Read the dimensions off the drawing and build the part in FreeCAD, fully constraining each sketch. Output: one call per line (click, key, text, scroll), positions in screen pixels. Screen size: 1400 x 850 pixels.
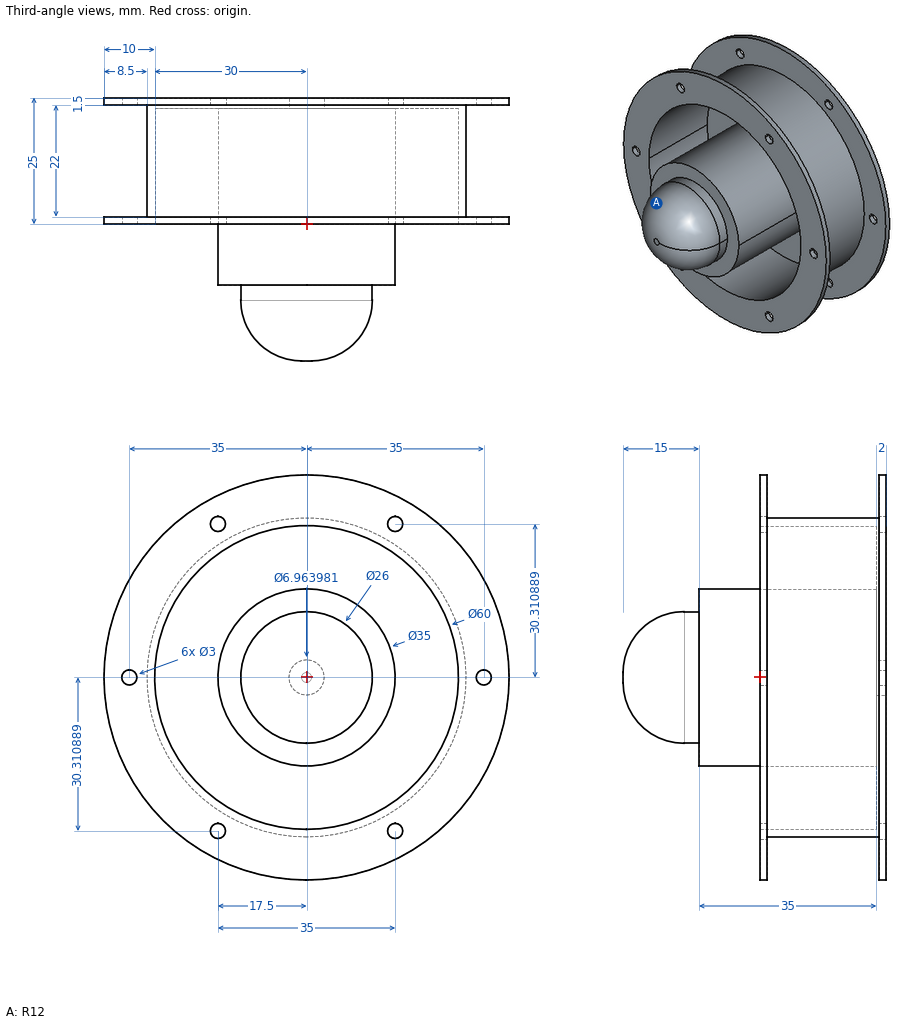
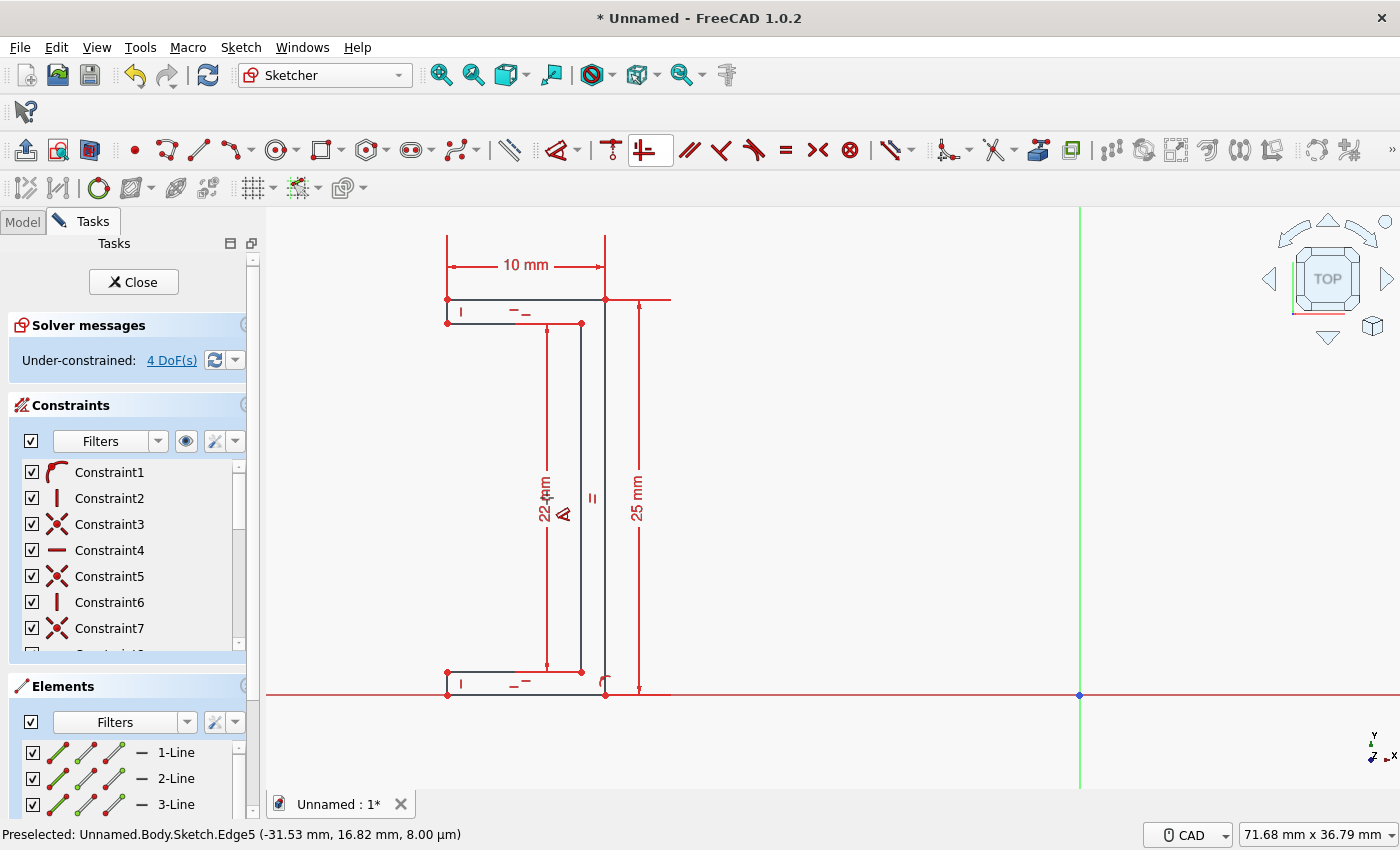
click(494, 695)
click(526, 729)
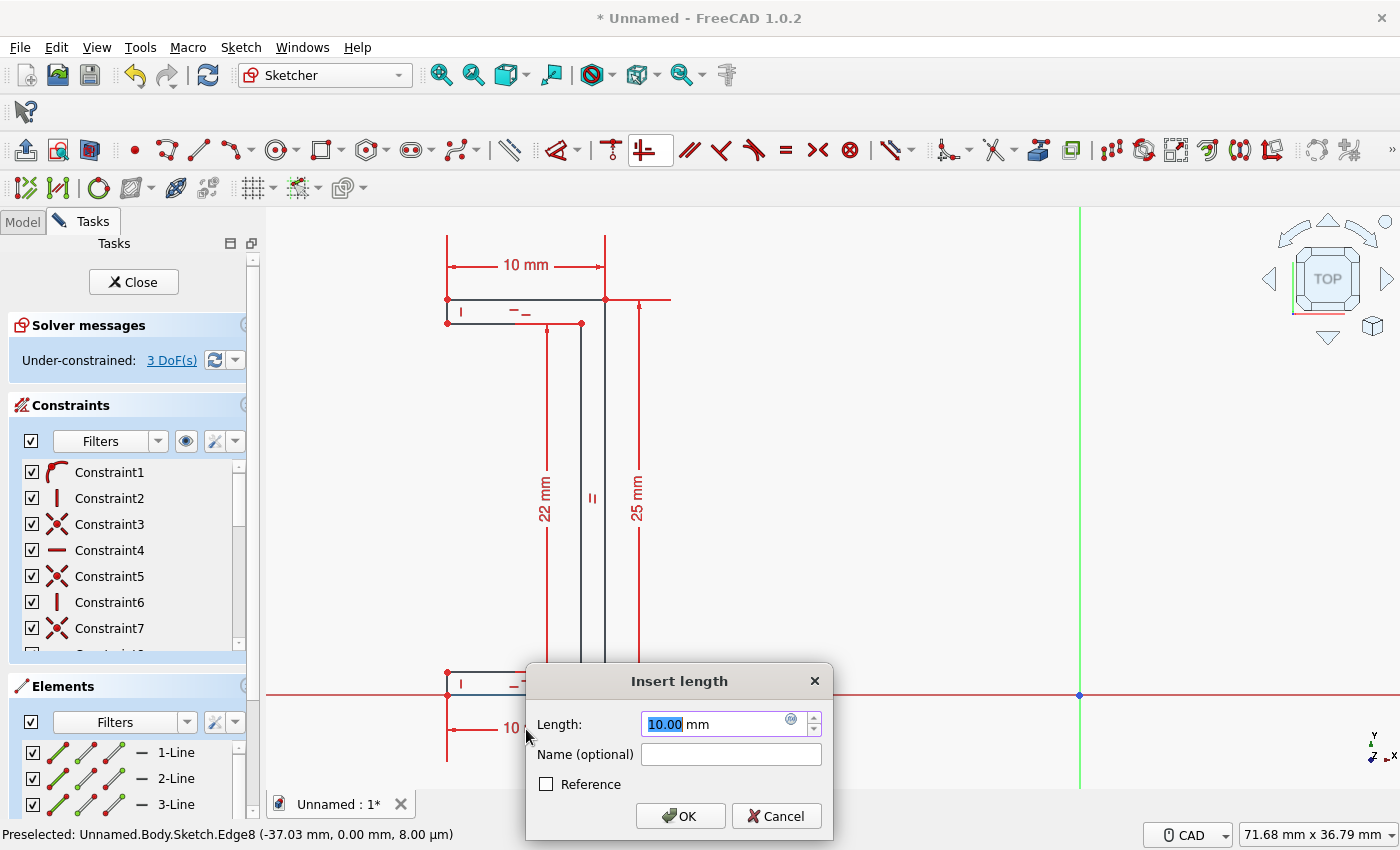
text(10)
key(Return)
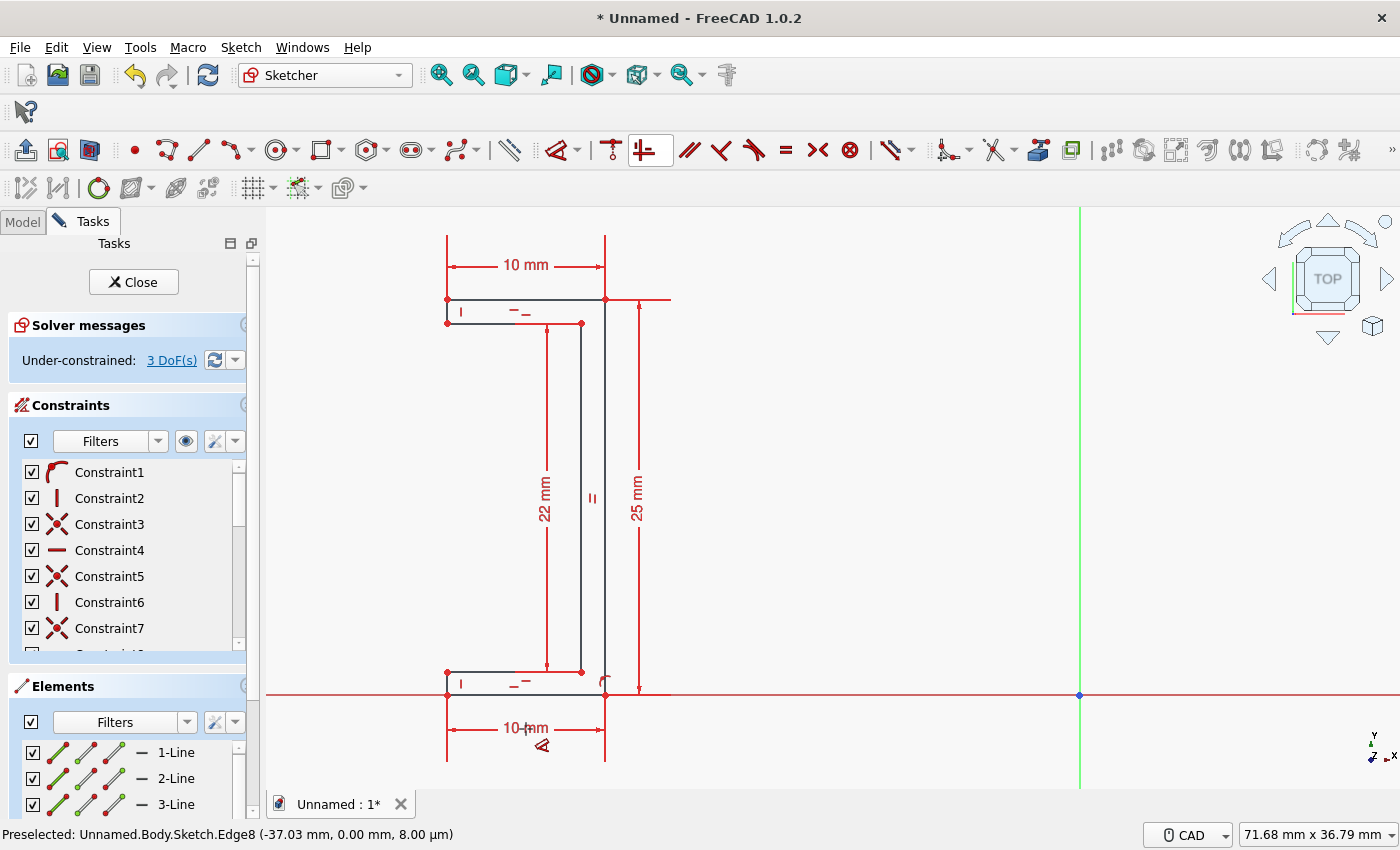
scroll(447, 309, up, 3)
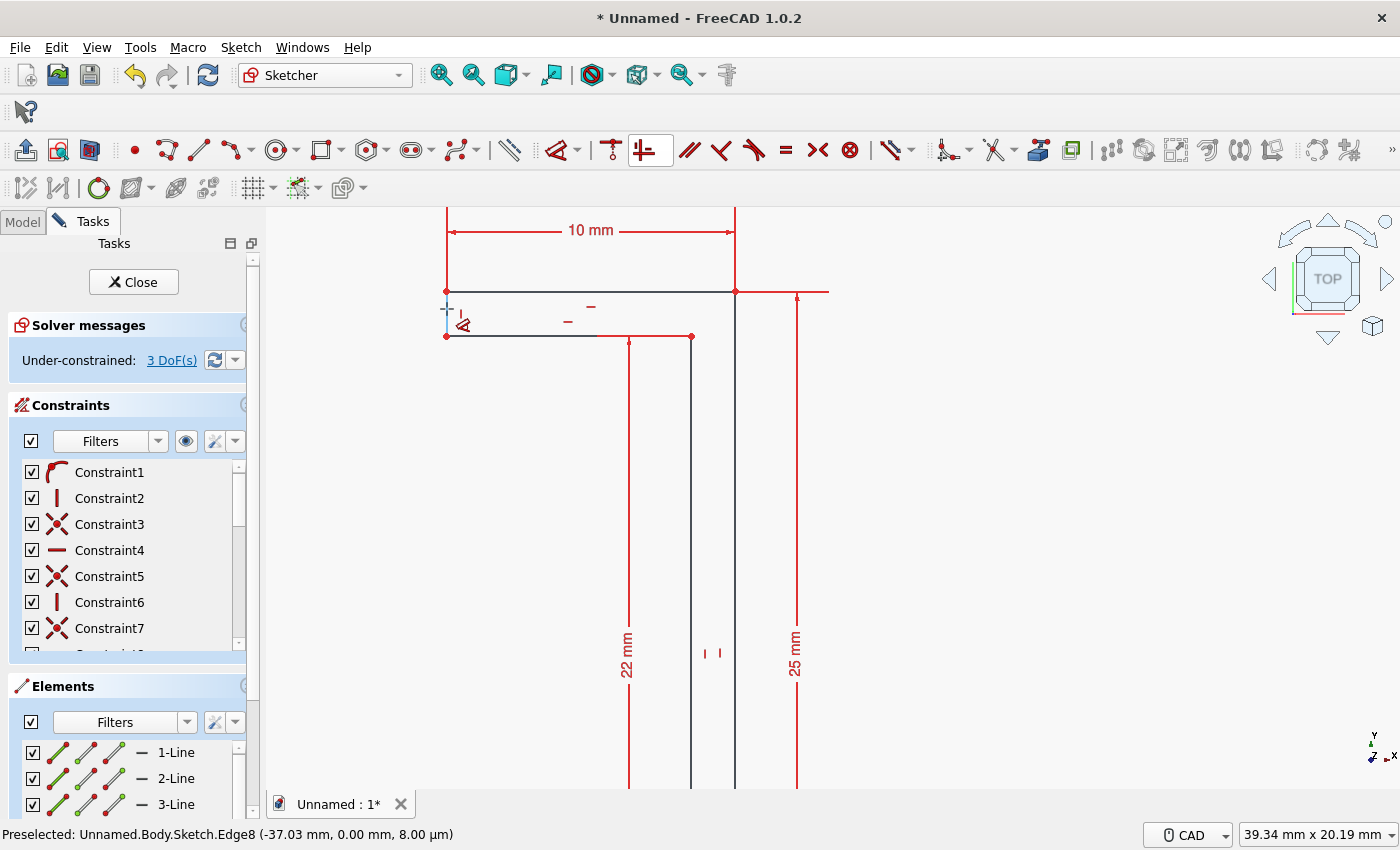
click(447, 309)
click(413, 314)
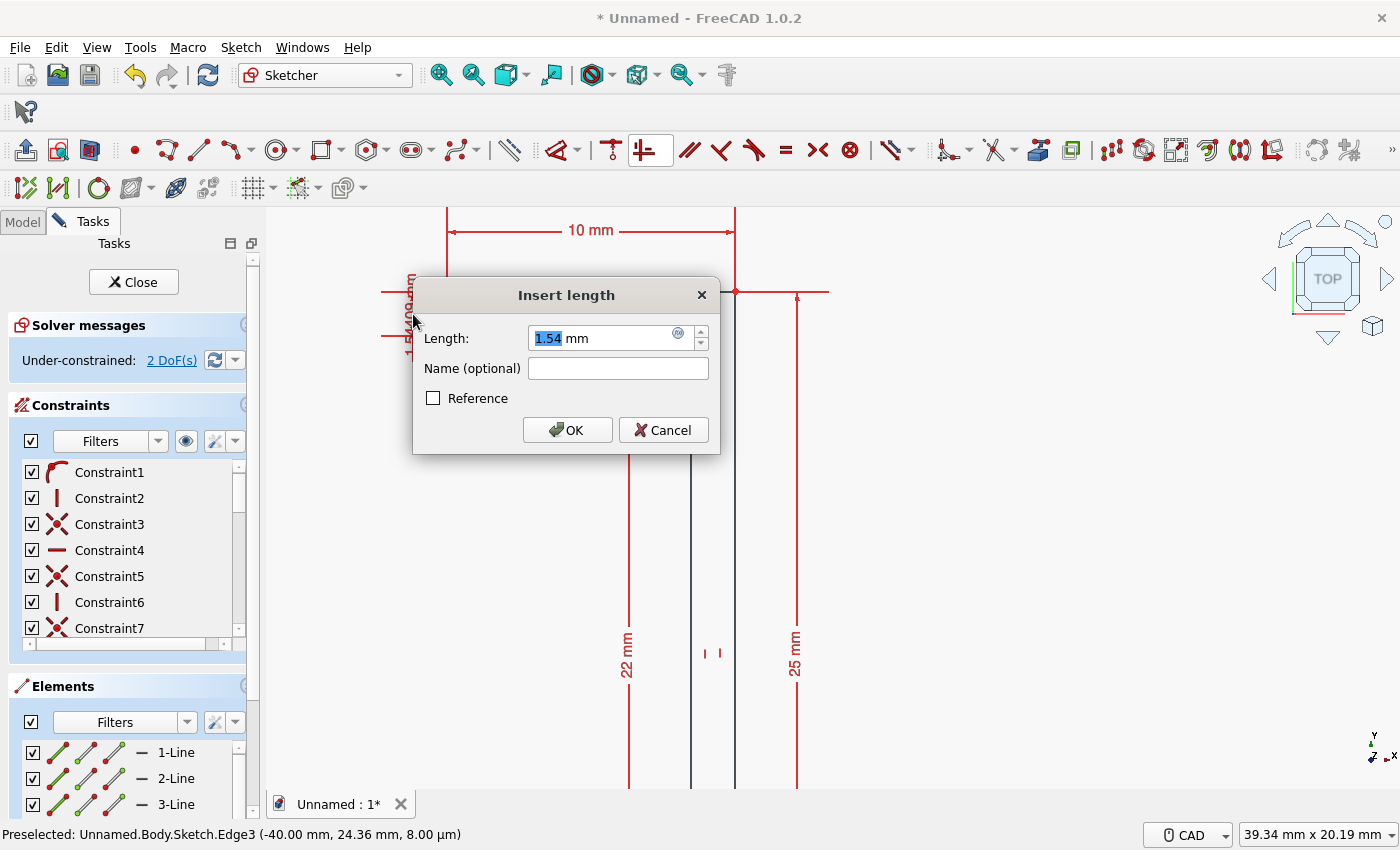
text(1.5)
key(Return)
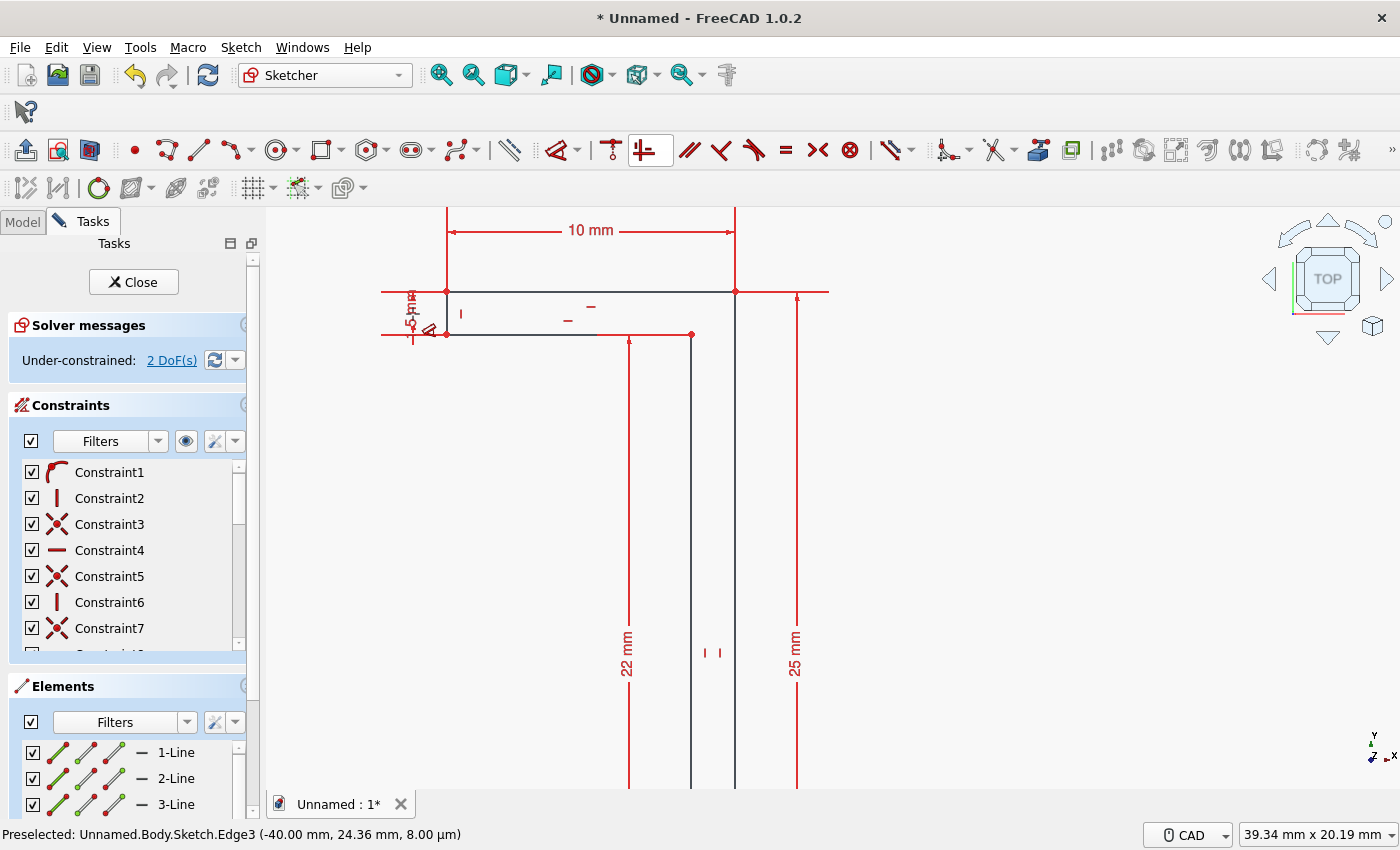
click(520, 335)
click(569, 369)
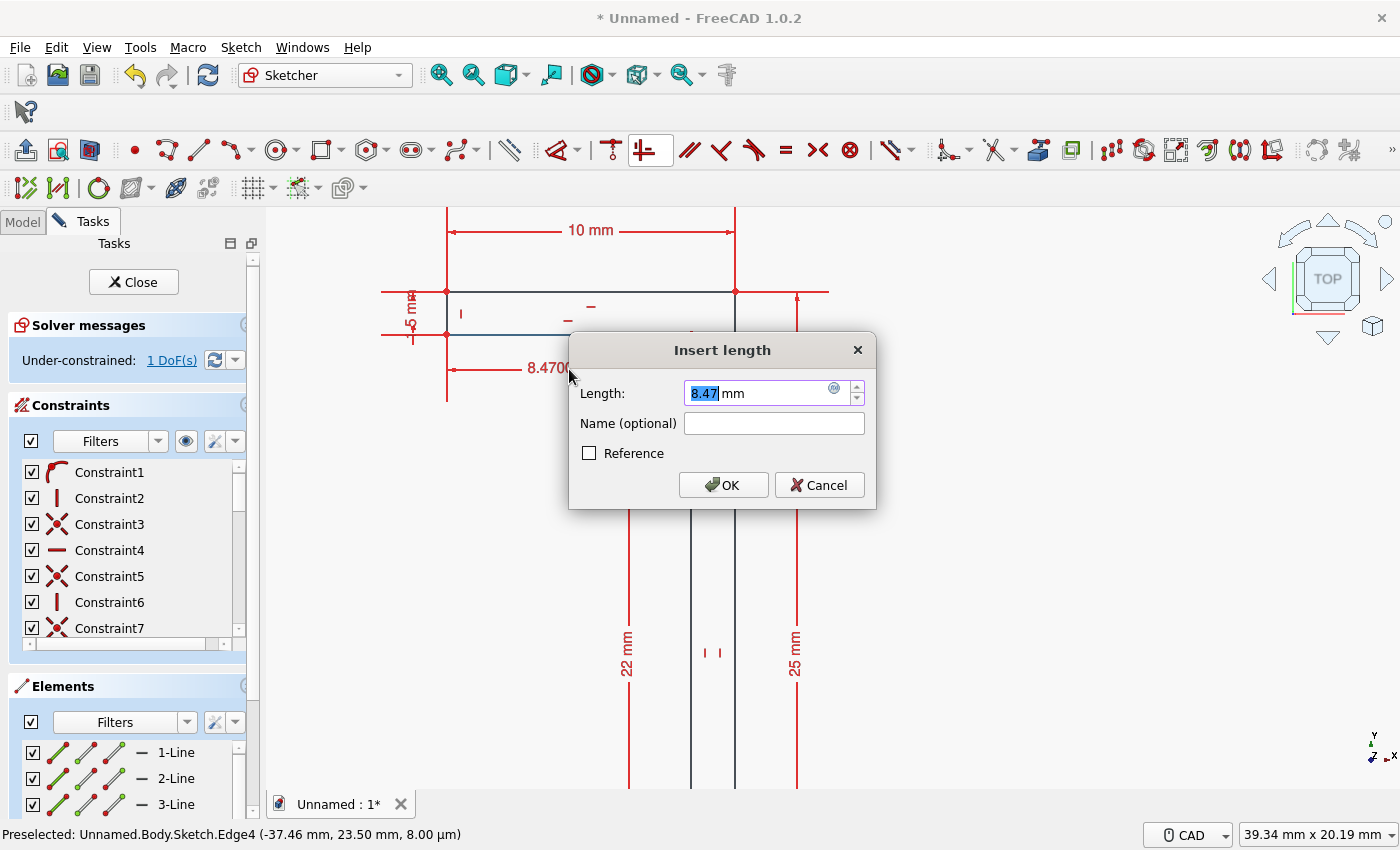
text(8.5)
key(Return)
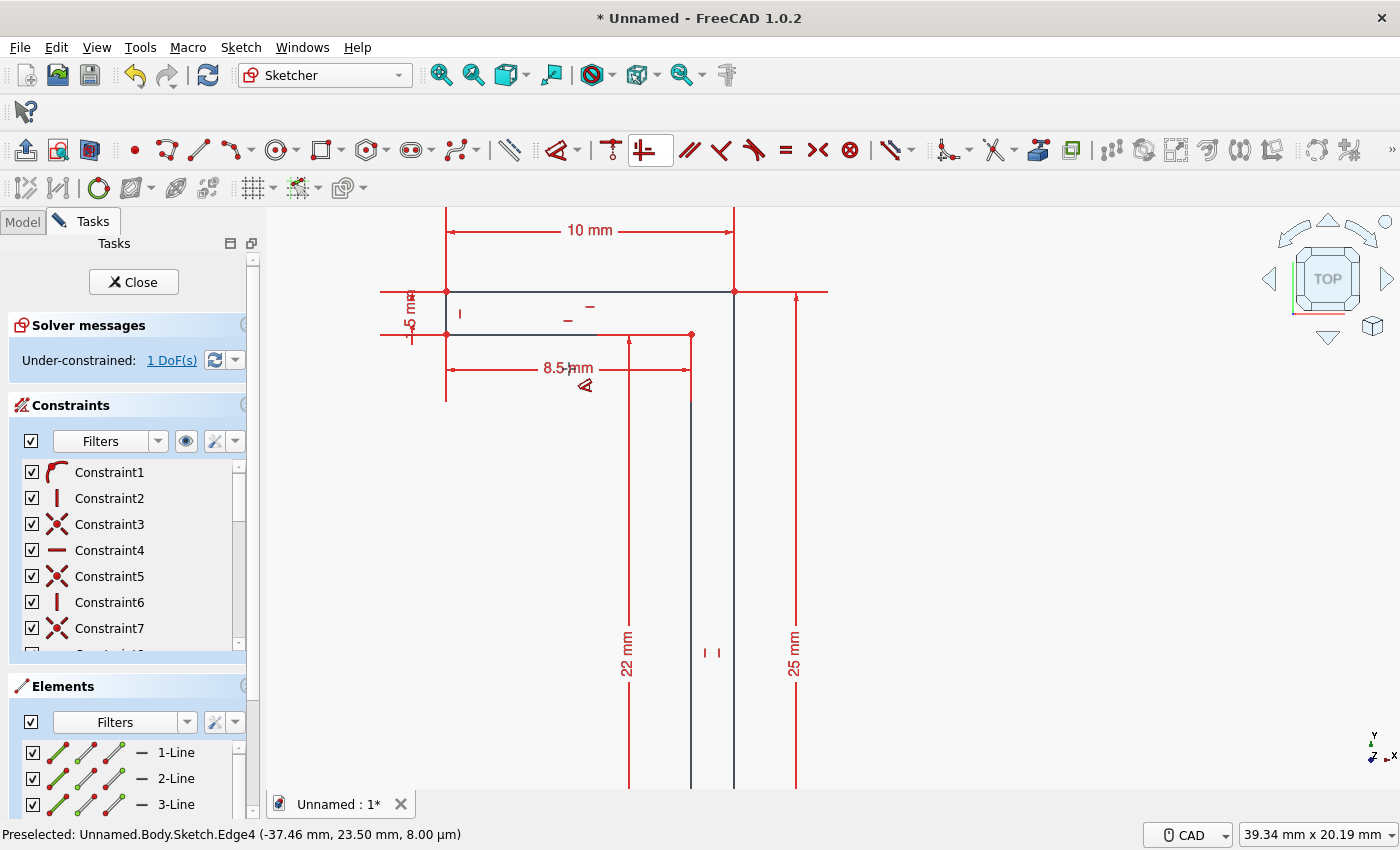
scroll(450, 311, down, 3)